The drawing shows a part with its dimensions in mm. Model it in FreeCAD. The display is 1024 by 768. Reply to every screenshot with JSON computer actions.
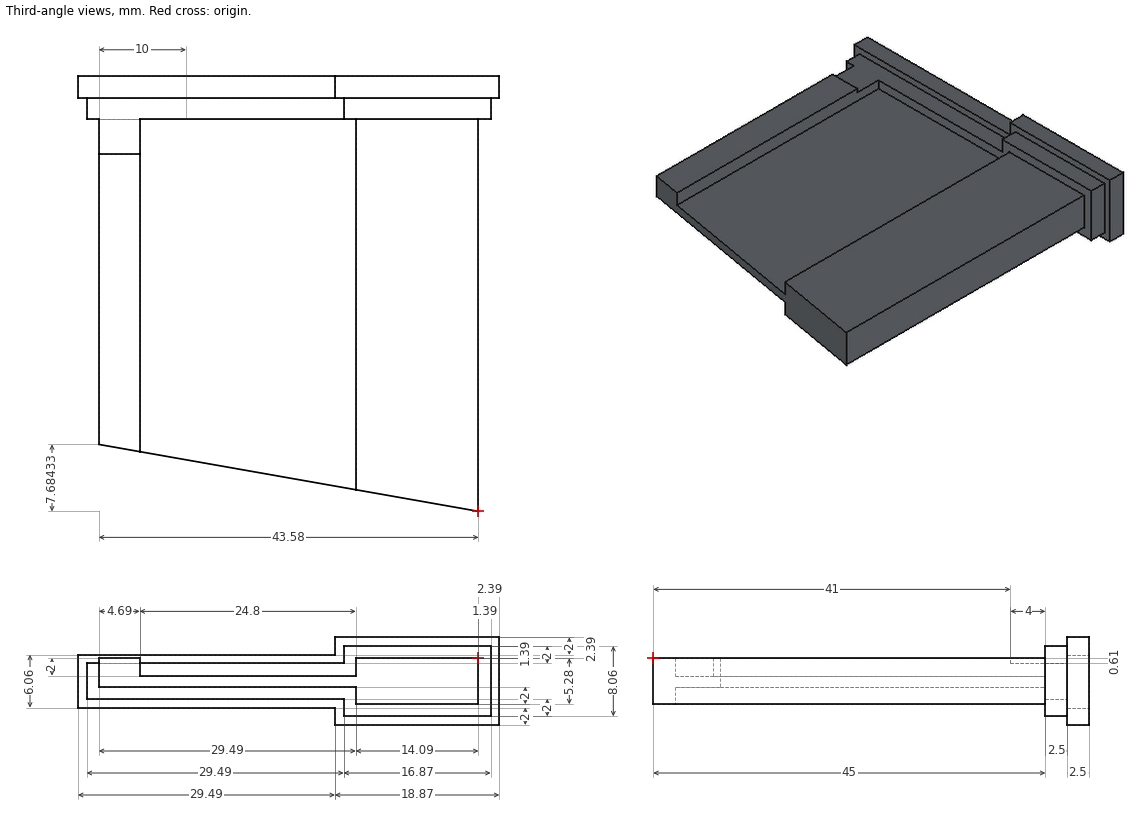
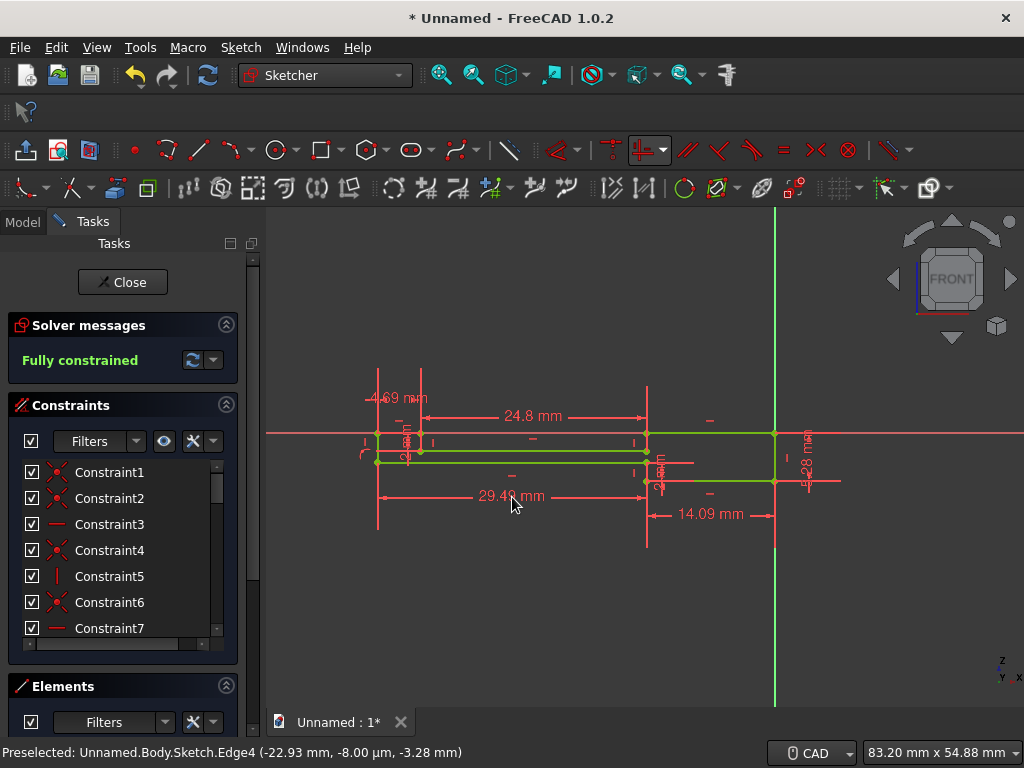
{"action": "left_click", "coordinate": [123, 282]}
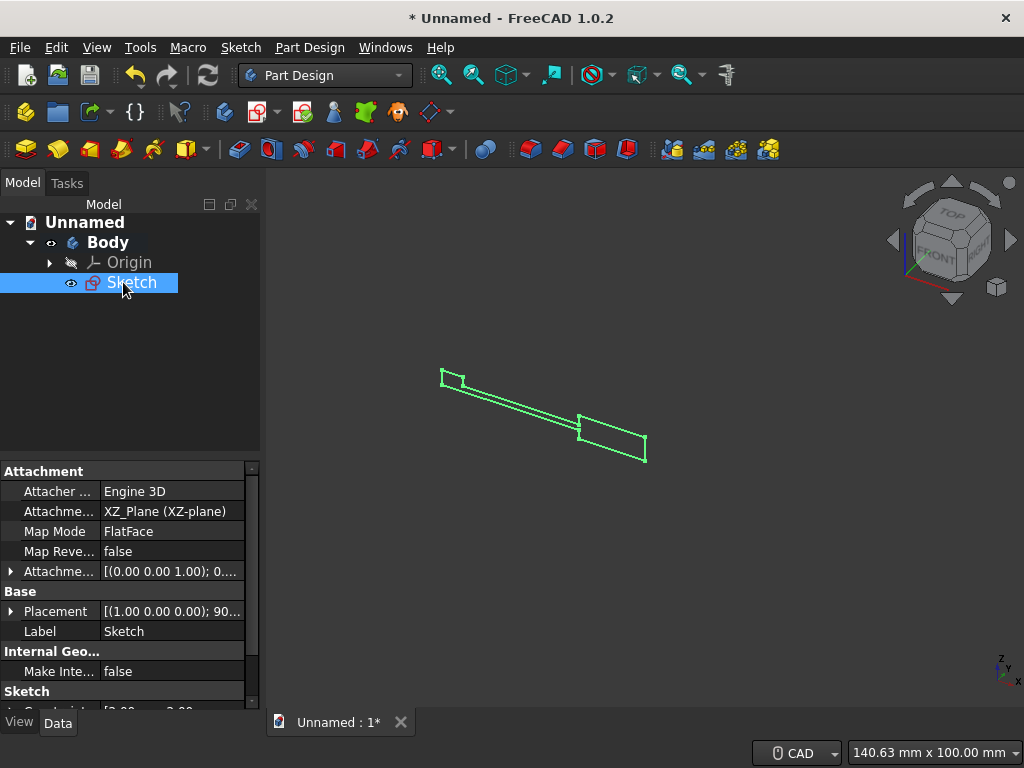
{"action": "left_click", "coordinate": [26, 150]}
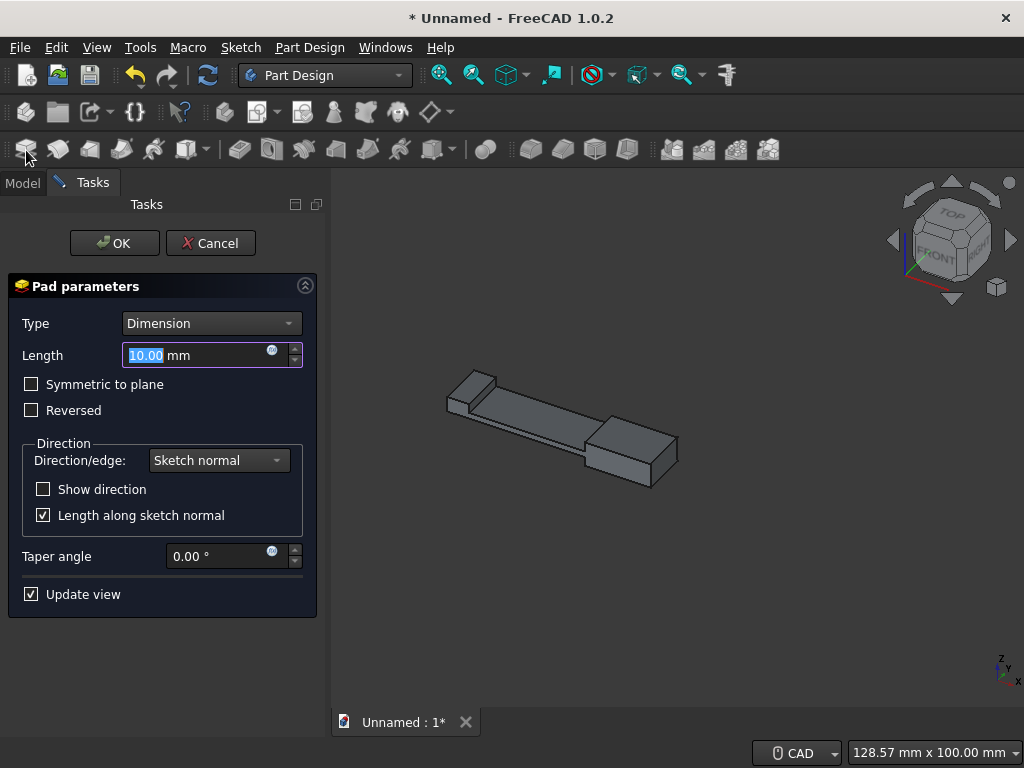
{"action": "type", "text": "45"}
{"action": "key", "text": "Tab"}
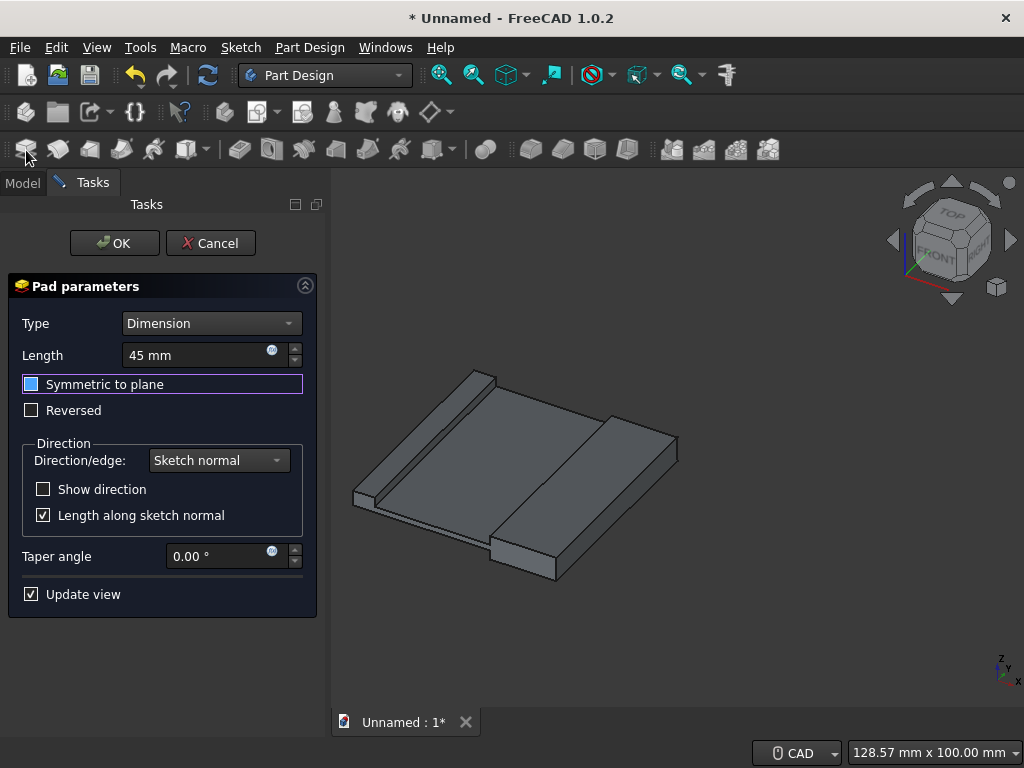
{"action": "left_click", "coordinate": [30, 410]}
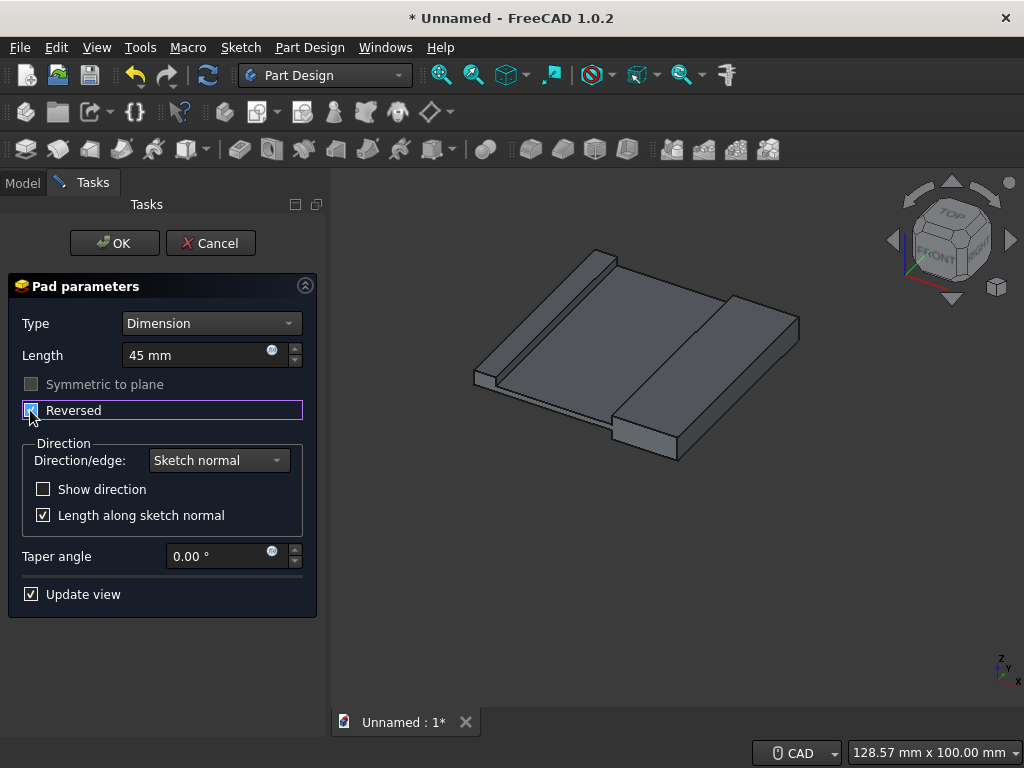
{"action": "left_click", "coordinate": [115, 243]}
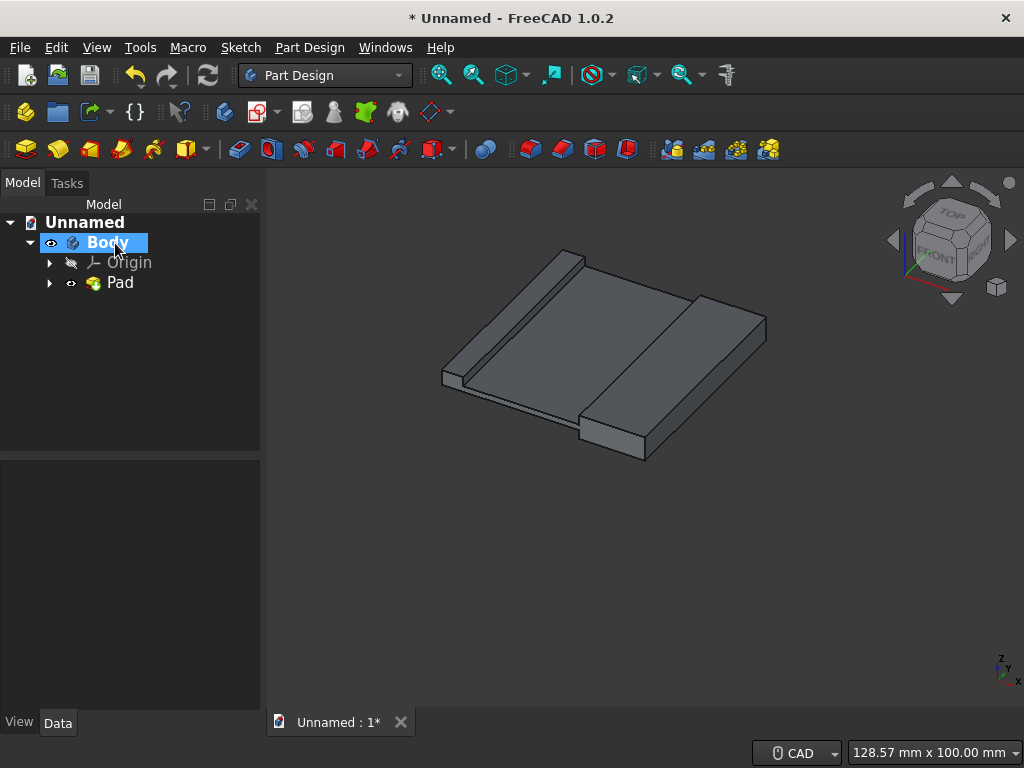
{"action": "key", "text": "v f"}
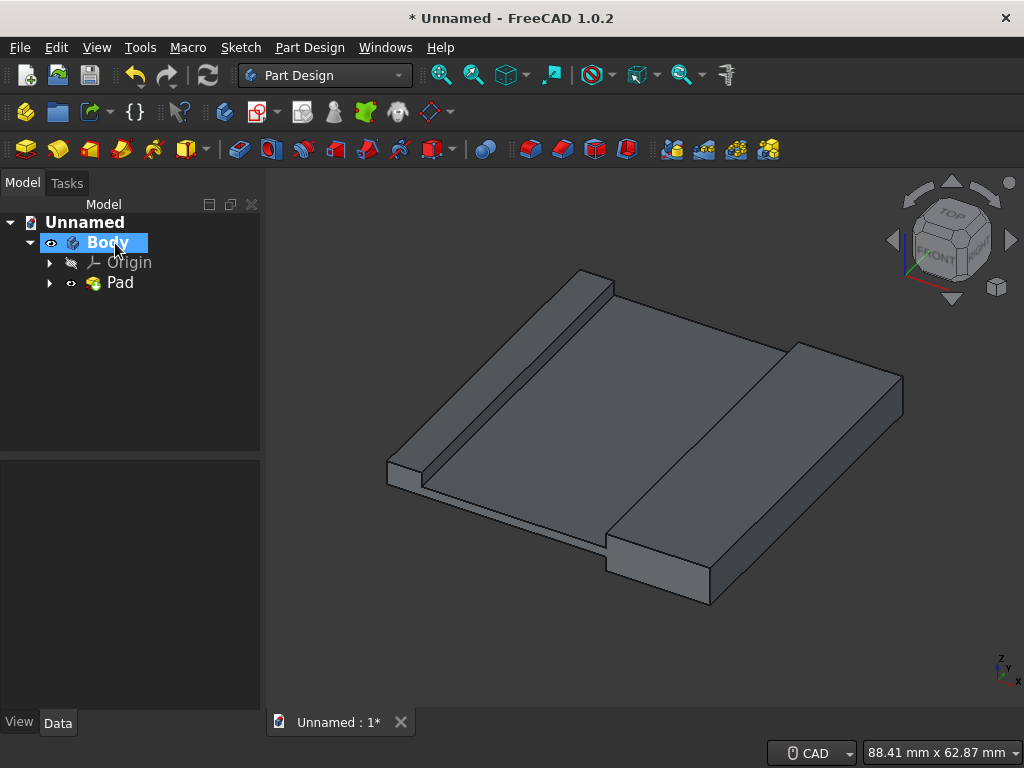
{"action": "left_click", "coordinate": [810, 399]}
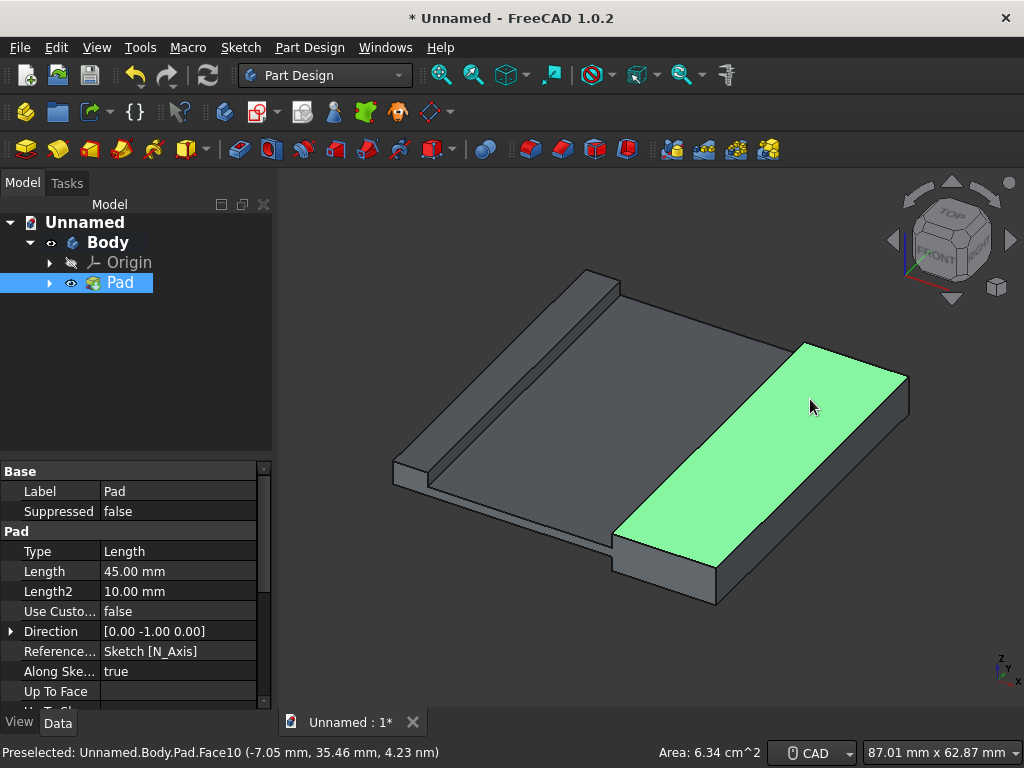
{"action": "left_click", "coordinate": [258, 112]}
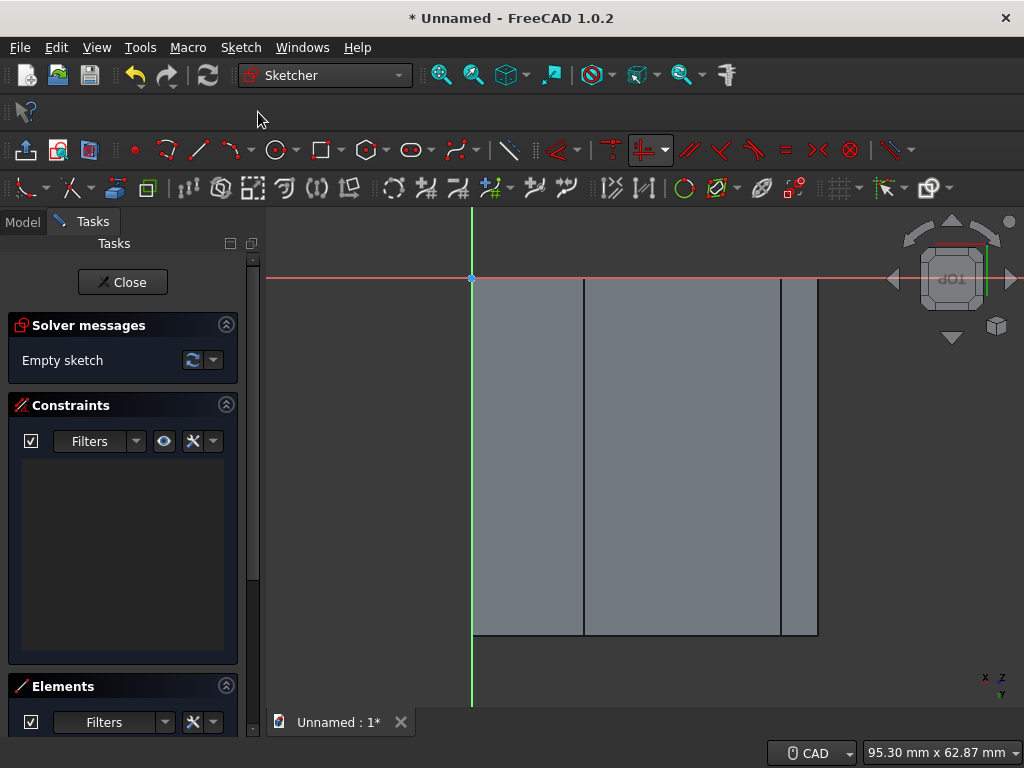
{"action": "left_click", "coordinate": [168, 150]}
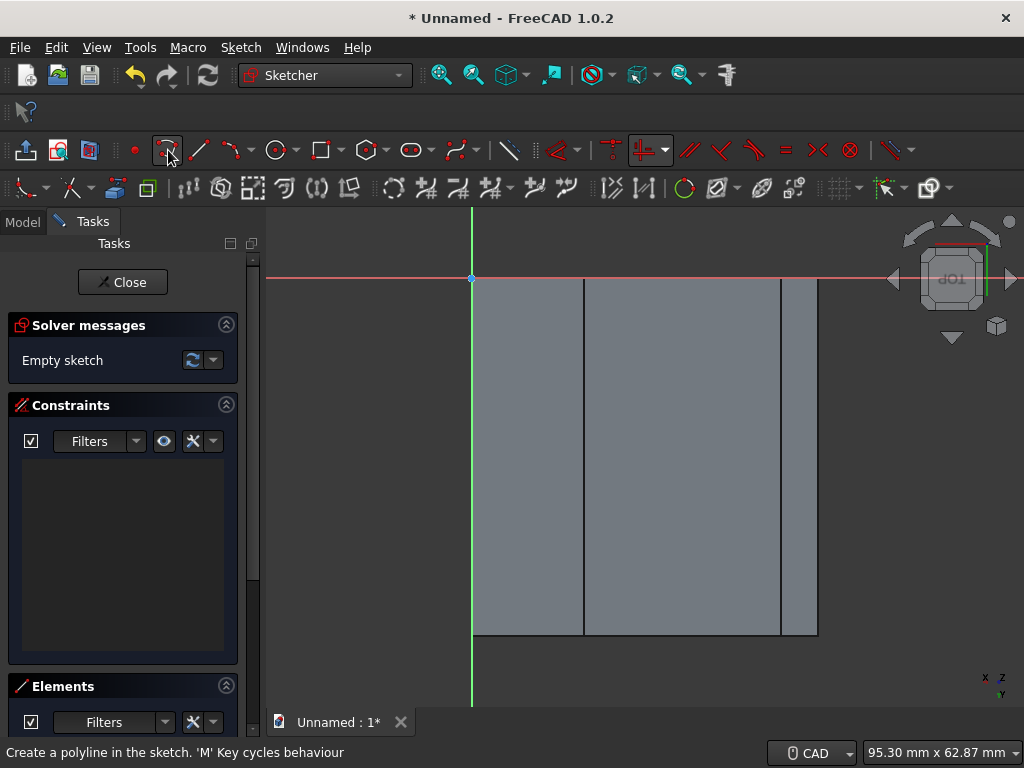
{"action": "left_click", "coordinate": [472, 278]}
{"action": "left_click", "coordinate": [818, 339]}
{"action": "left_click", "coordinate": [818, 287]}
{"action": "left_click", "coordinate": [472, 278]}
{"action": "key", "text": "Escape"}
{"action": "key", "text": "Escape"}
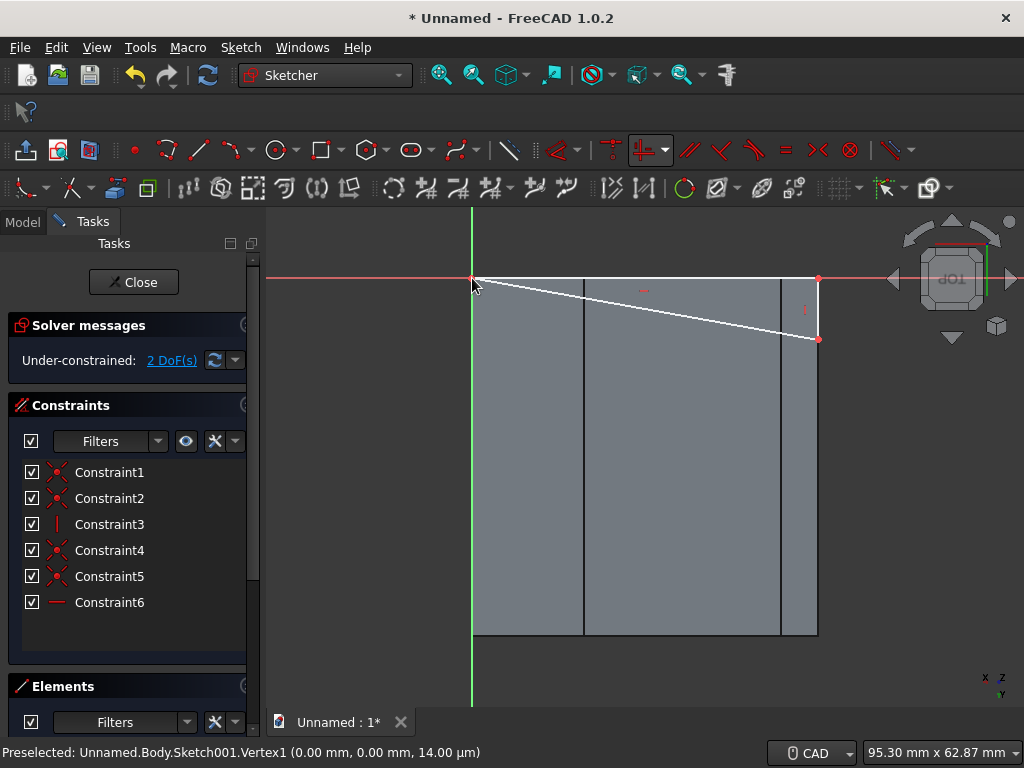
{"action": "left_click", "coordinate": [556, 150]}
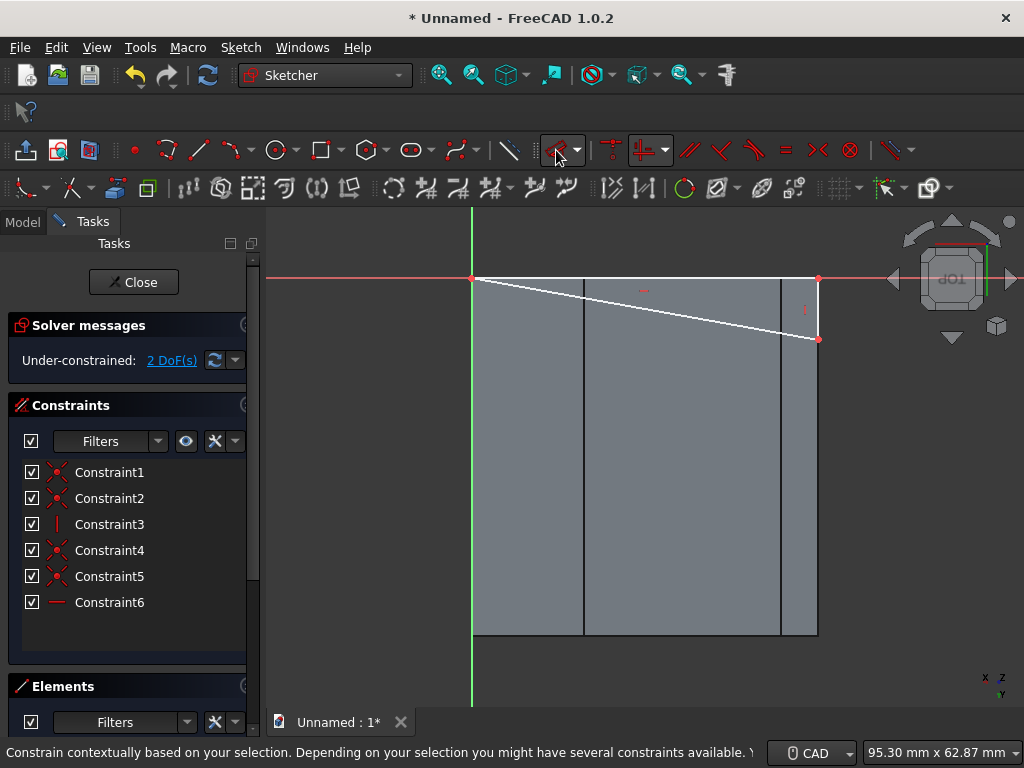
{"action": "left_click", "coordinate": [714, 278]}
{"action": "left_click", "coordinate": [645, 244]}